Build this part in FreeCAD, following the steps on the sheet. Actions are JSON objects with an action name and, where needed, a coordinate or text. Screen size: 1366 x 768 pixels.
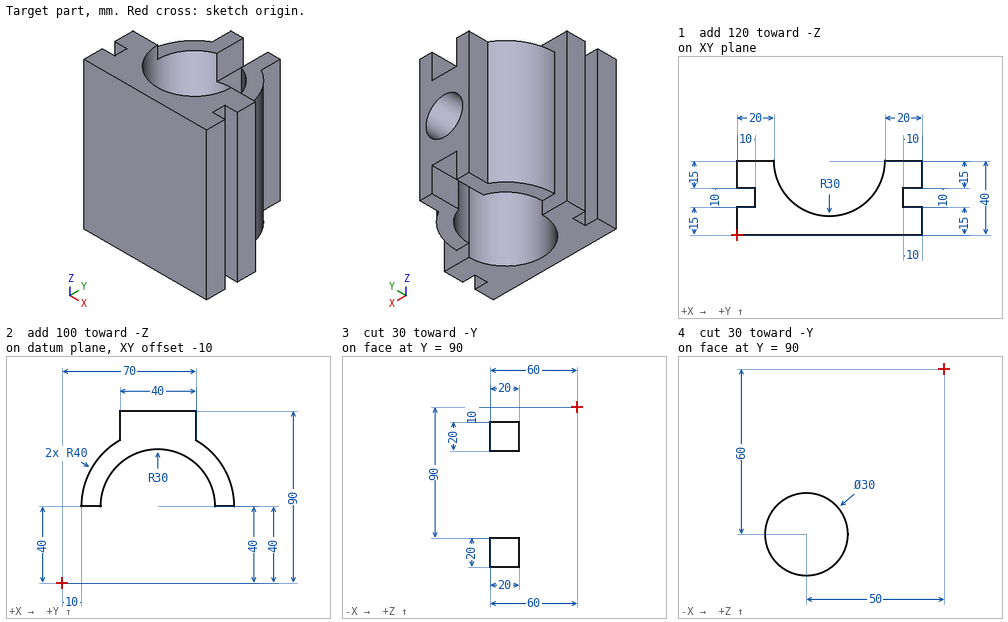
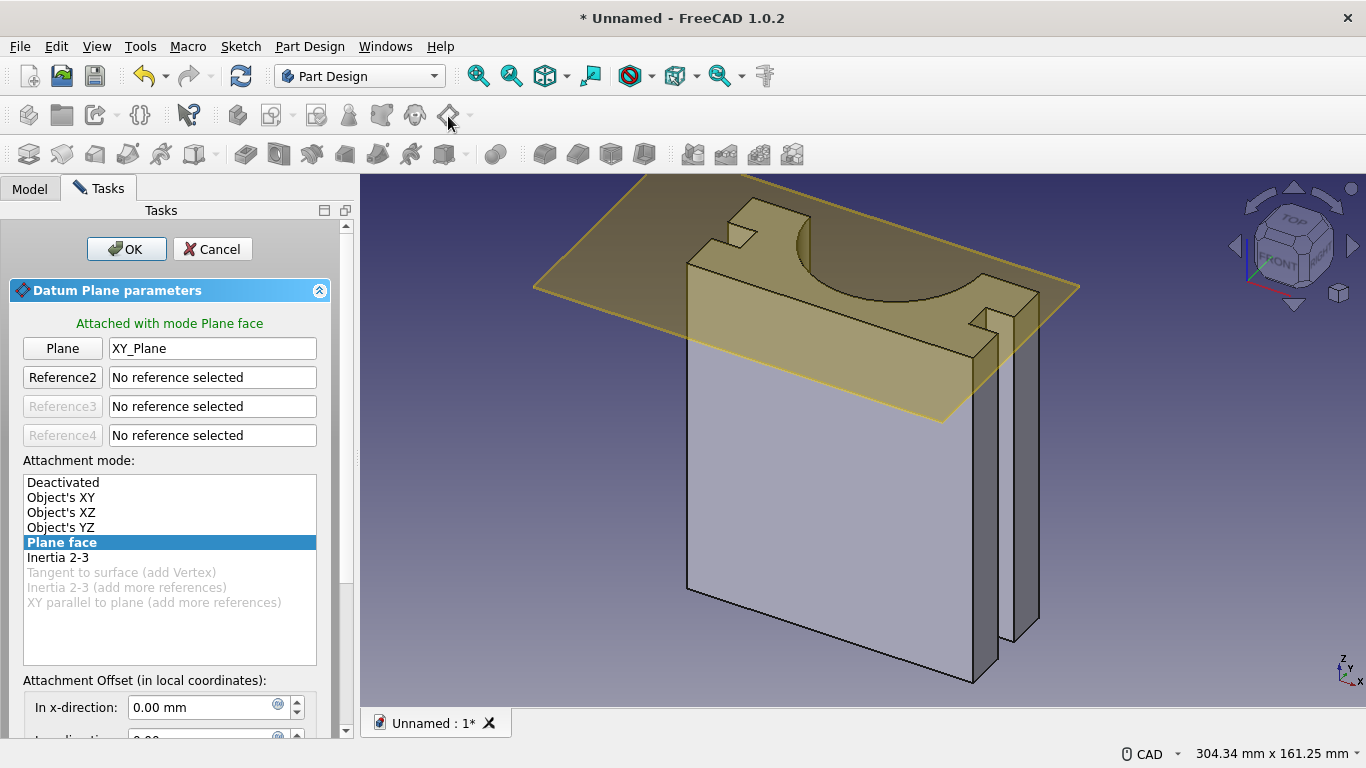
{"action": "scroll", "coordinate": [346, 479], "scroll_direction": "down", "scroll_amount": 2}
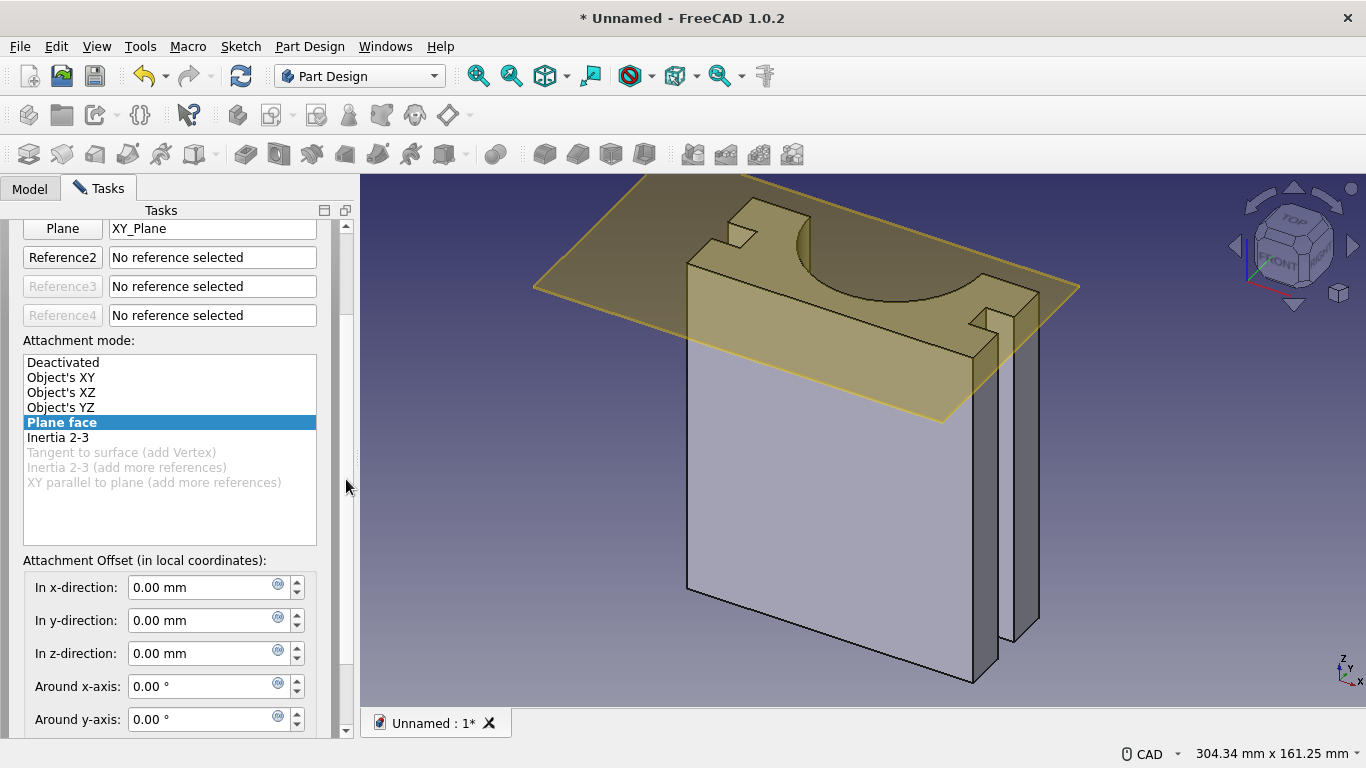
{"action": "triple_click", "coordinate": [210, 654]}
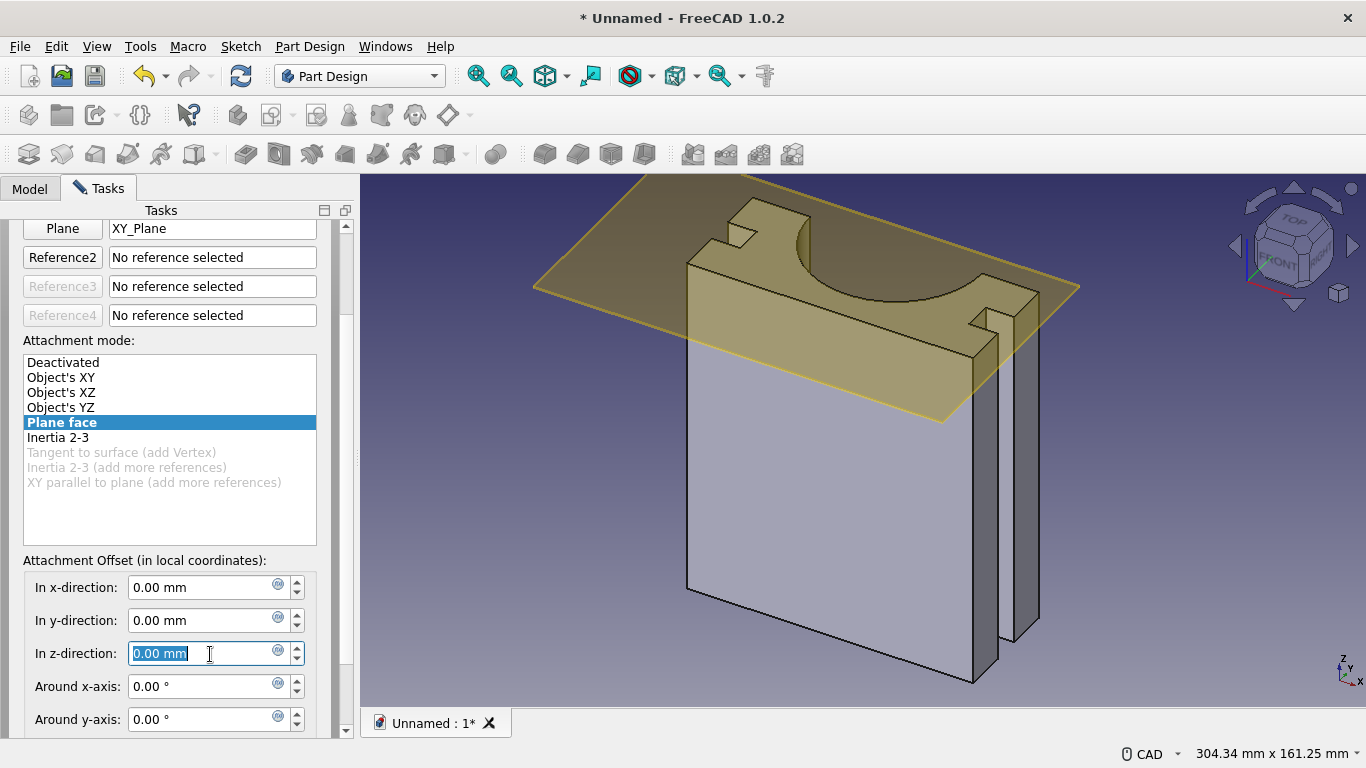
{"action": "type", "text": "-10"}
{"action": "key", "text": "Tab"}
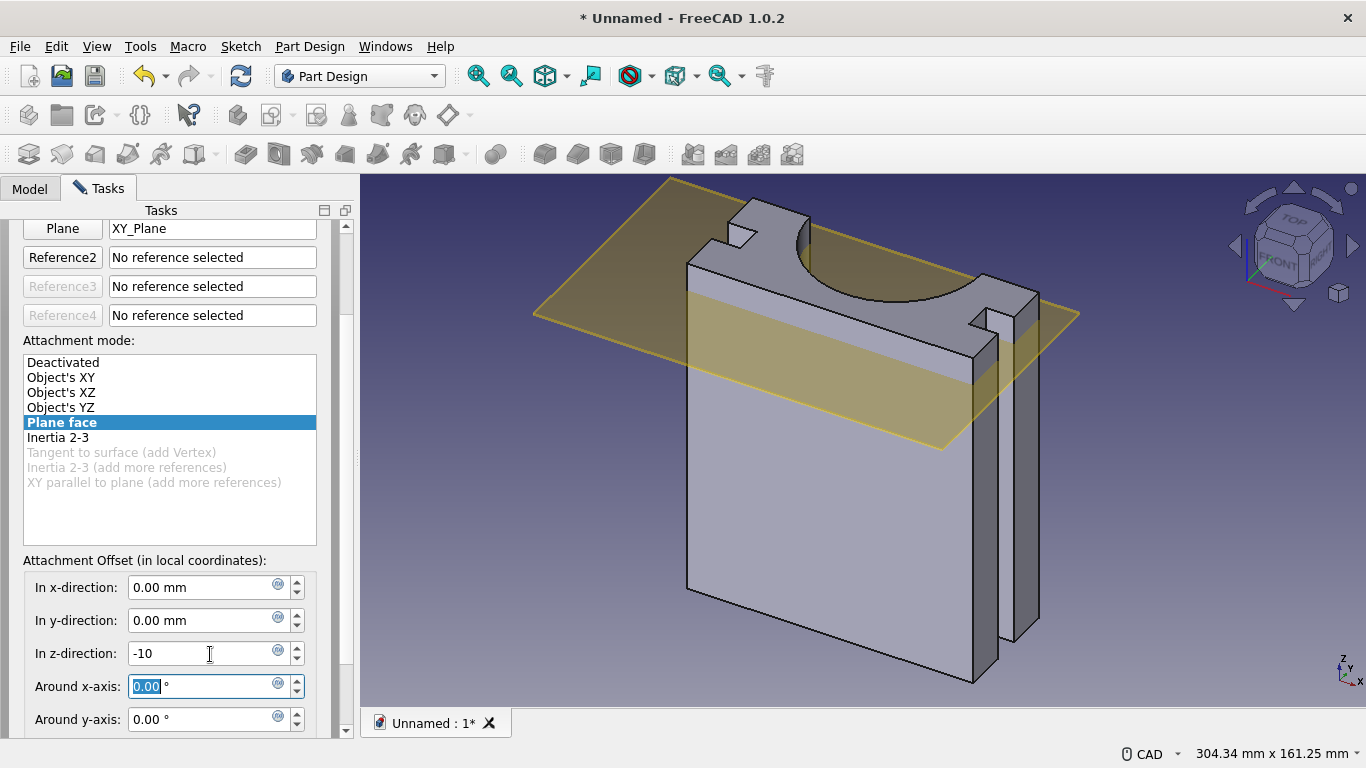
{"action": "scroll", "coordinate": [346, 479], "scroll_direction": "up", "scroll_amount": 3}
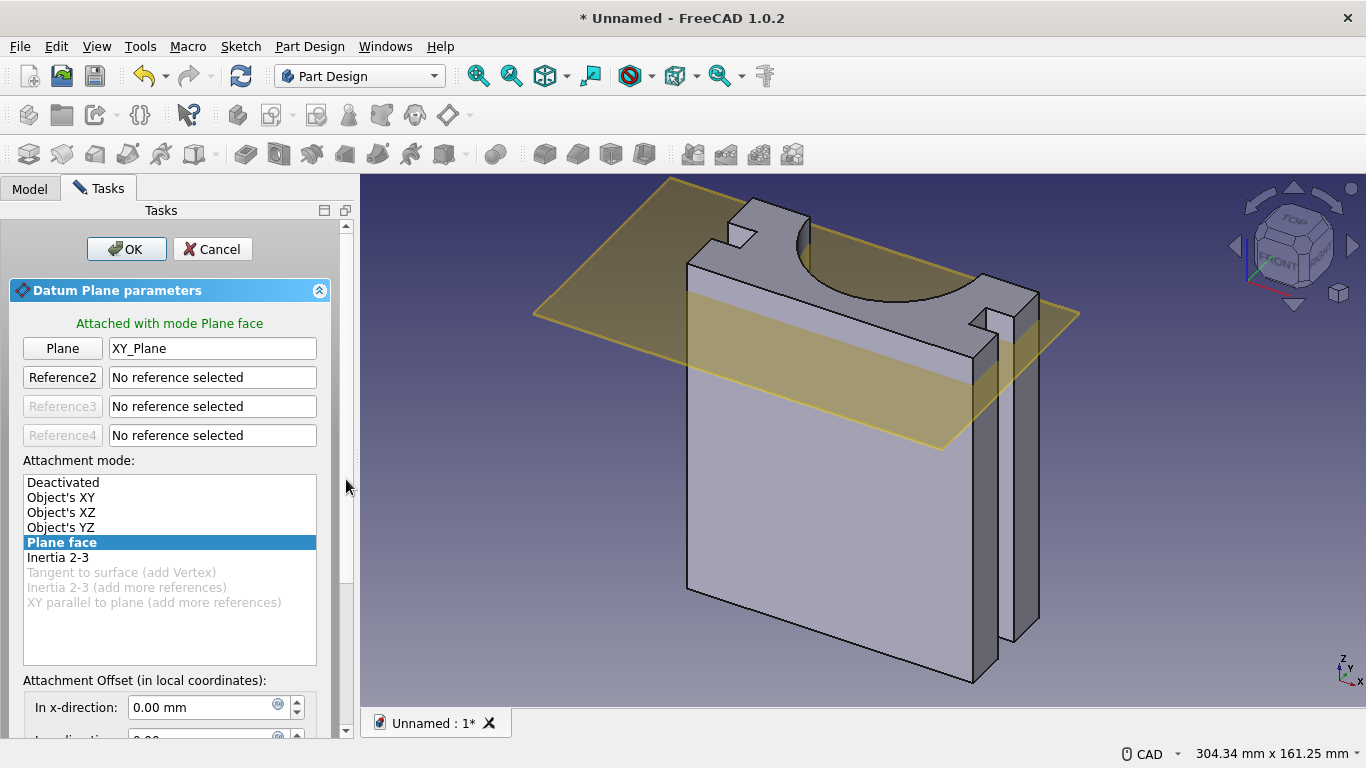
{"action": "left_click", "coordinate": [127, 249]}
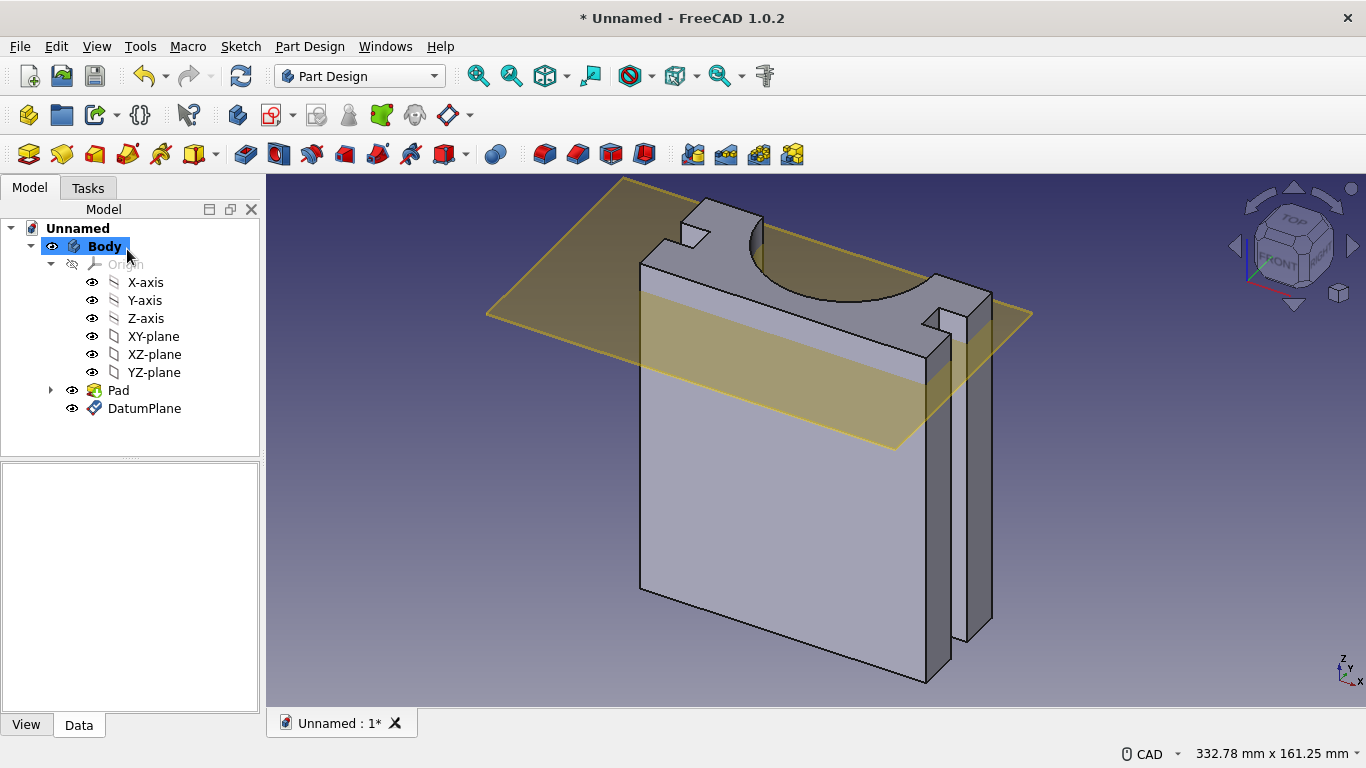
{"action": "left_click", "coordinate": [117, 408]}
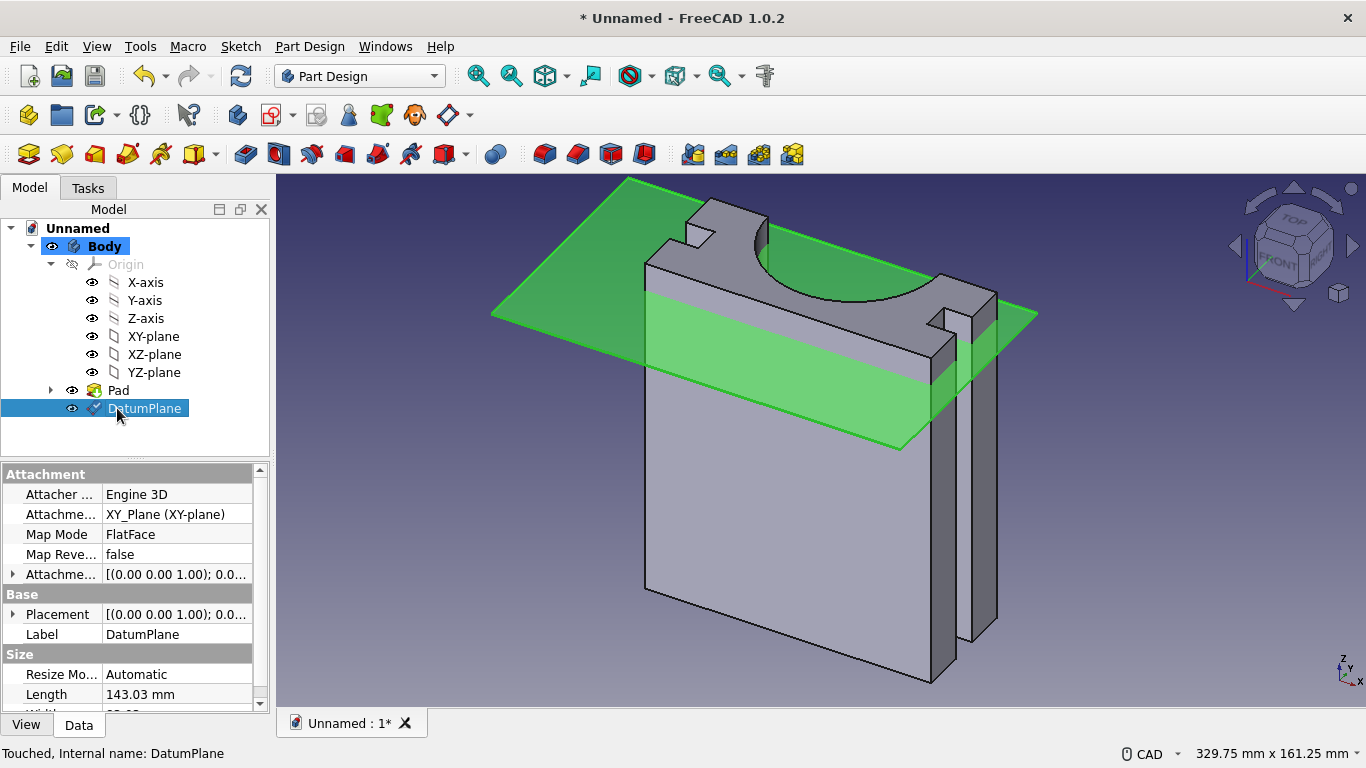
{"action": "left_click", "coordinate": [270, 116]}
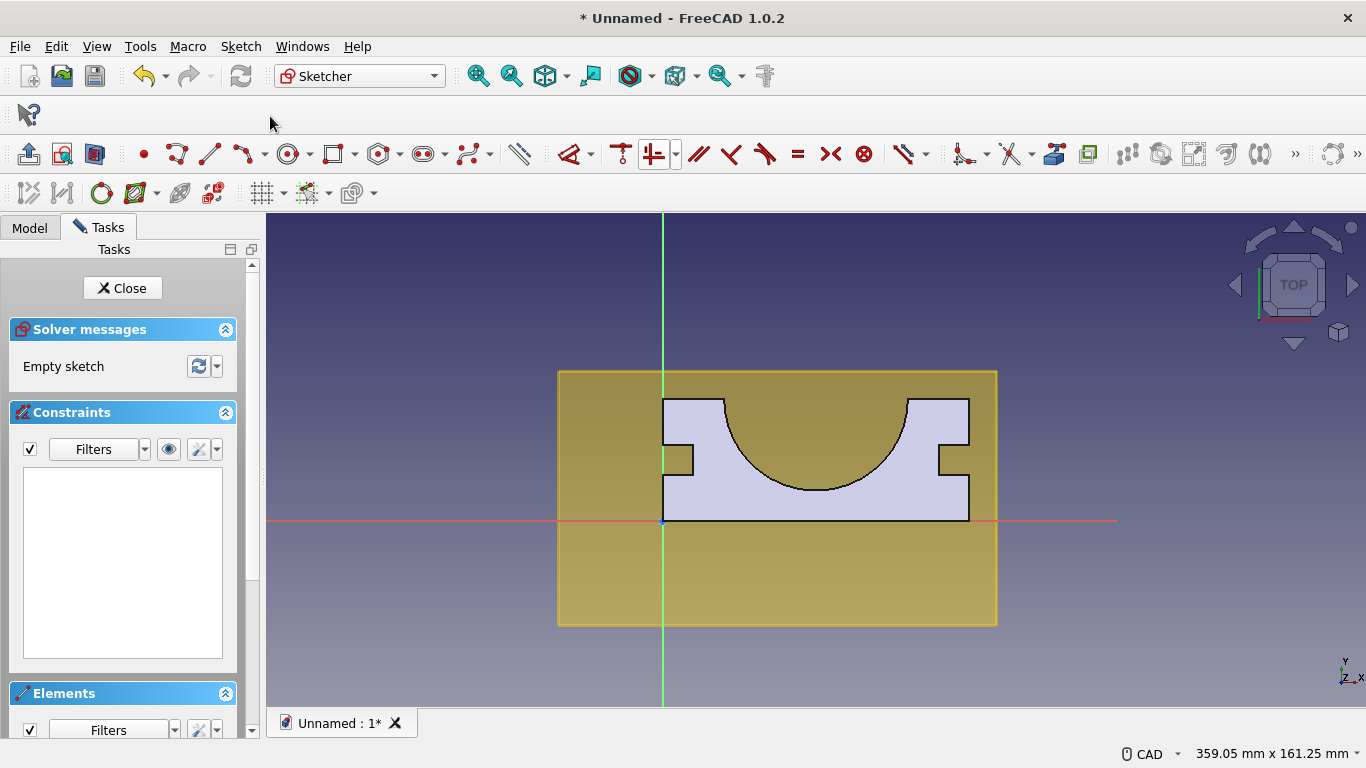
{"action": "left_click", "coordinate": [95, 154]}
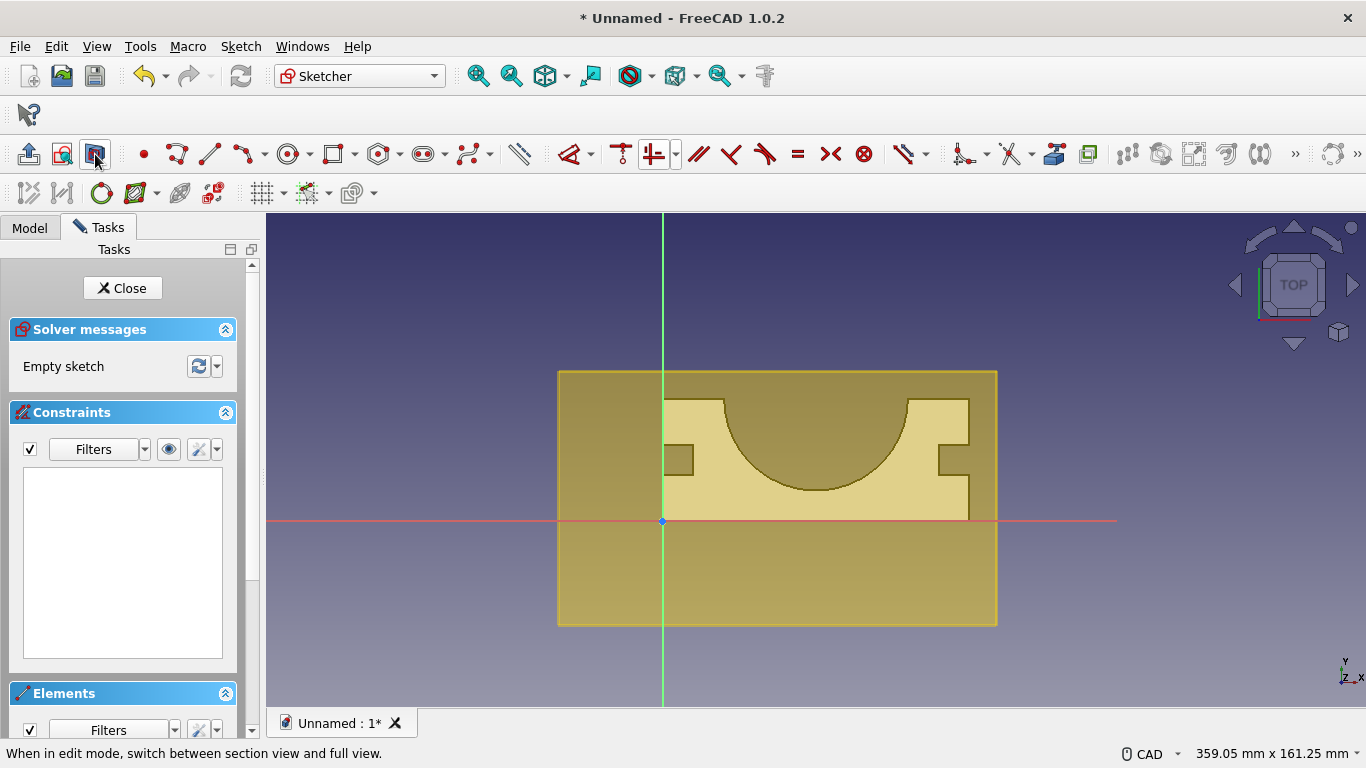
{"action": "scroll", "coordinate": [507, 679], "scroll_direction": "down", "scroll_amount": 1}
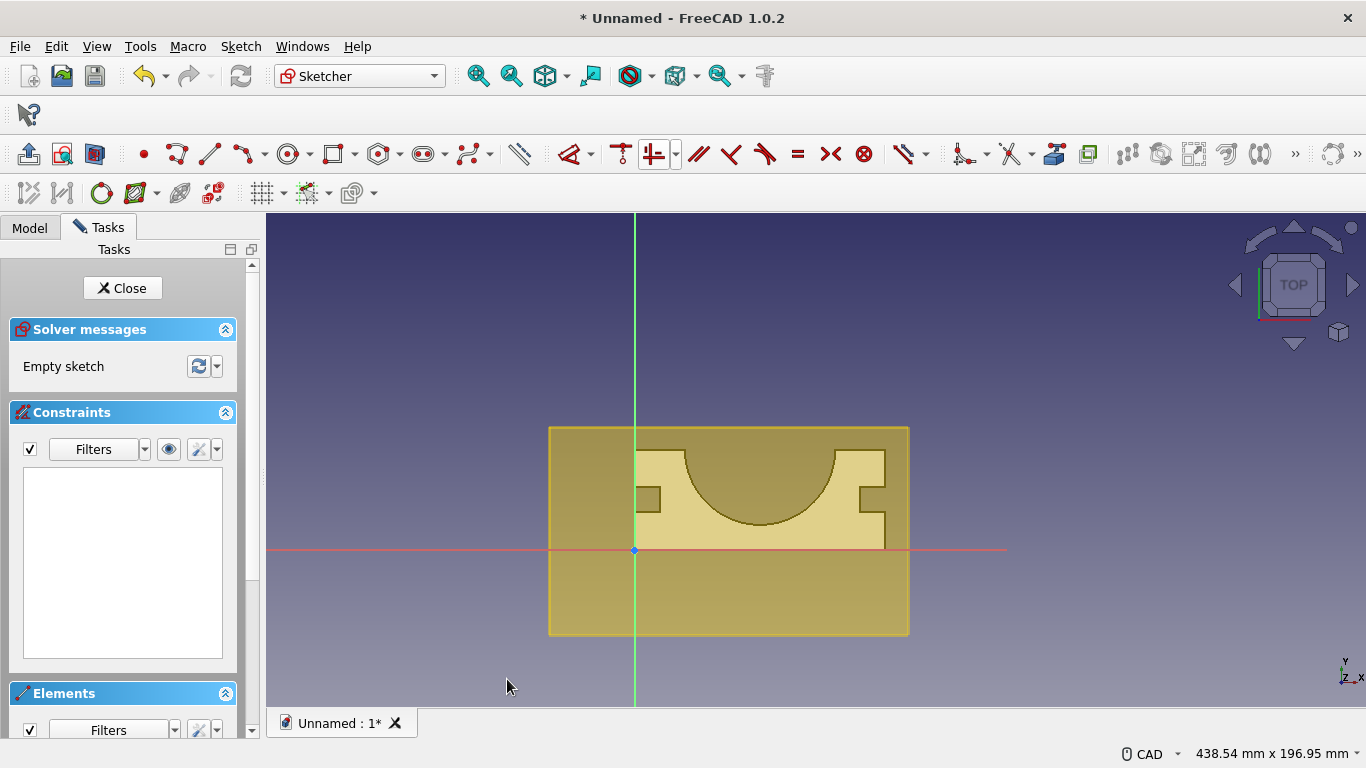
{"action": "scroll", "coordinate": [747, 391], "scroll_direction": "up", "scroll_amount": 2}